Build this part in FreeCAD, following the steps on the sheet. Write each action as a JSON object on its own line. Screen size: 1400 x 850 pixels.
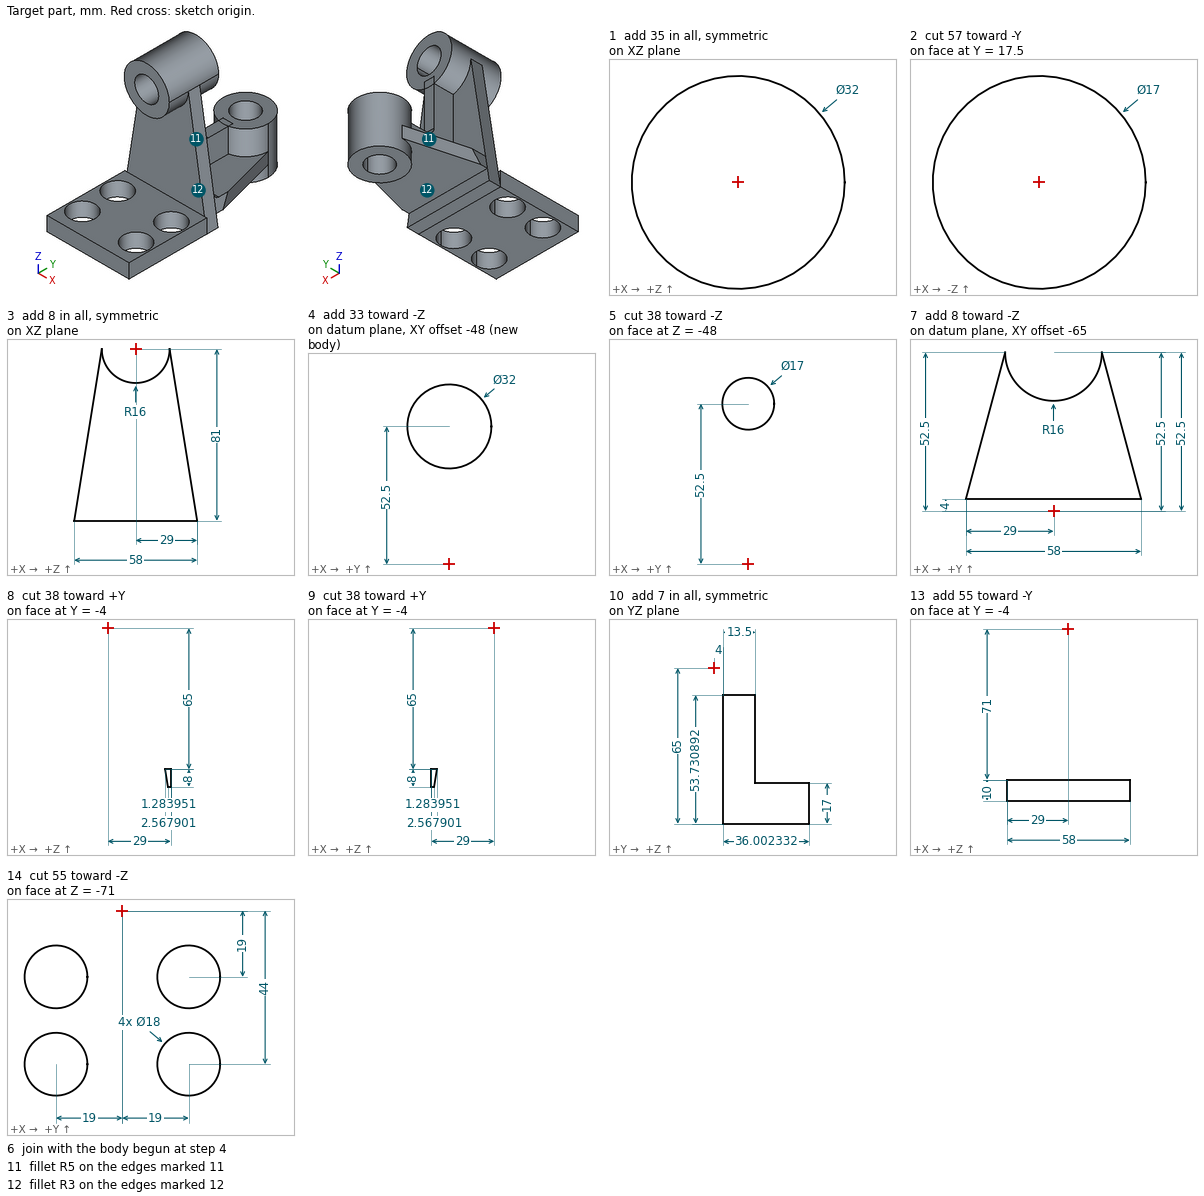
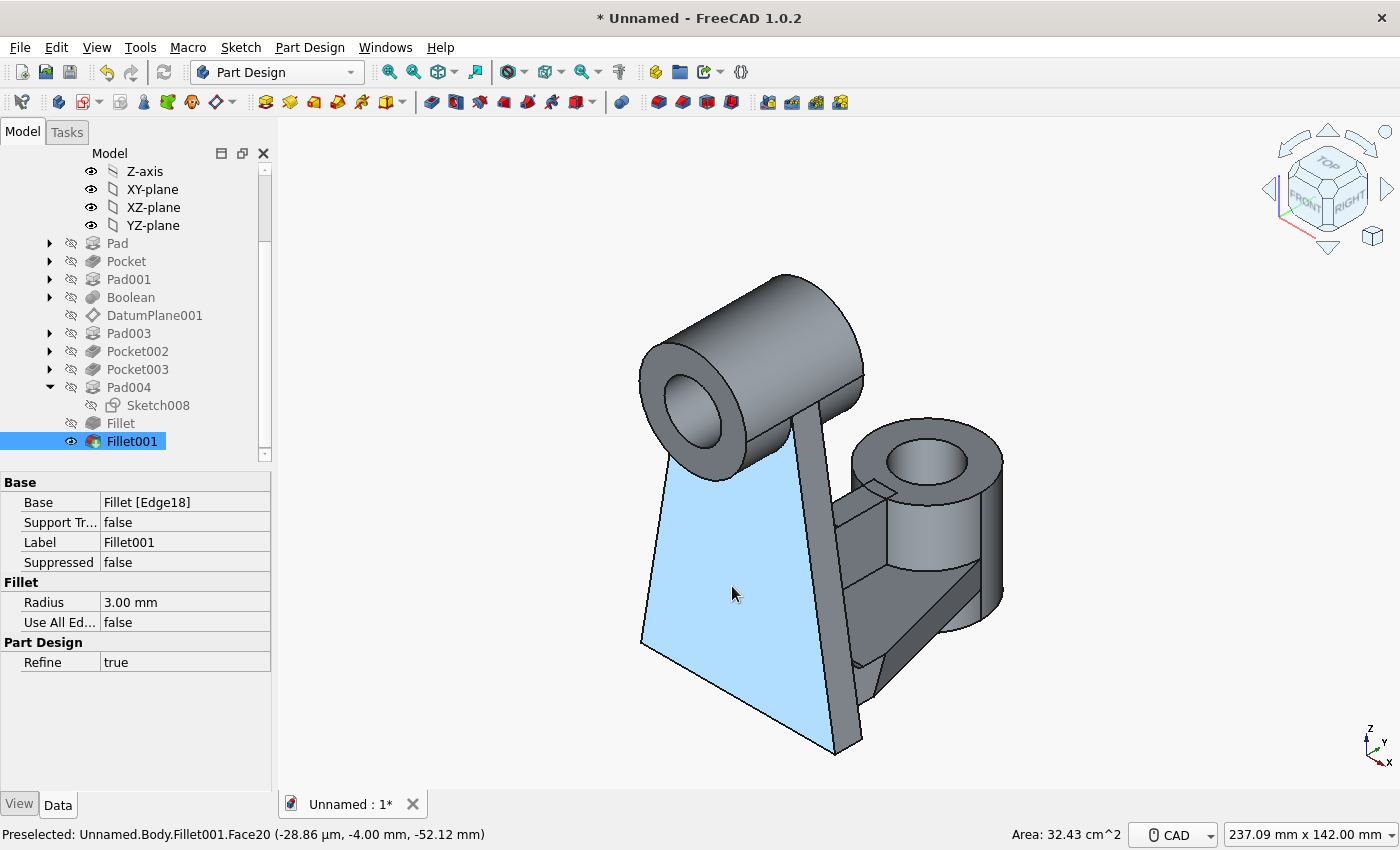
{"action": "left_click", "coordinate": [84, 102]}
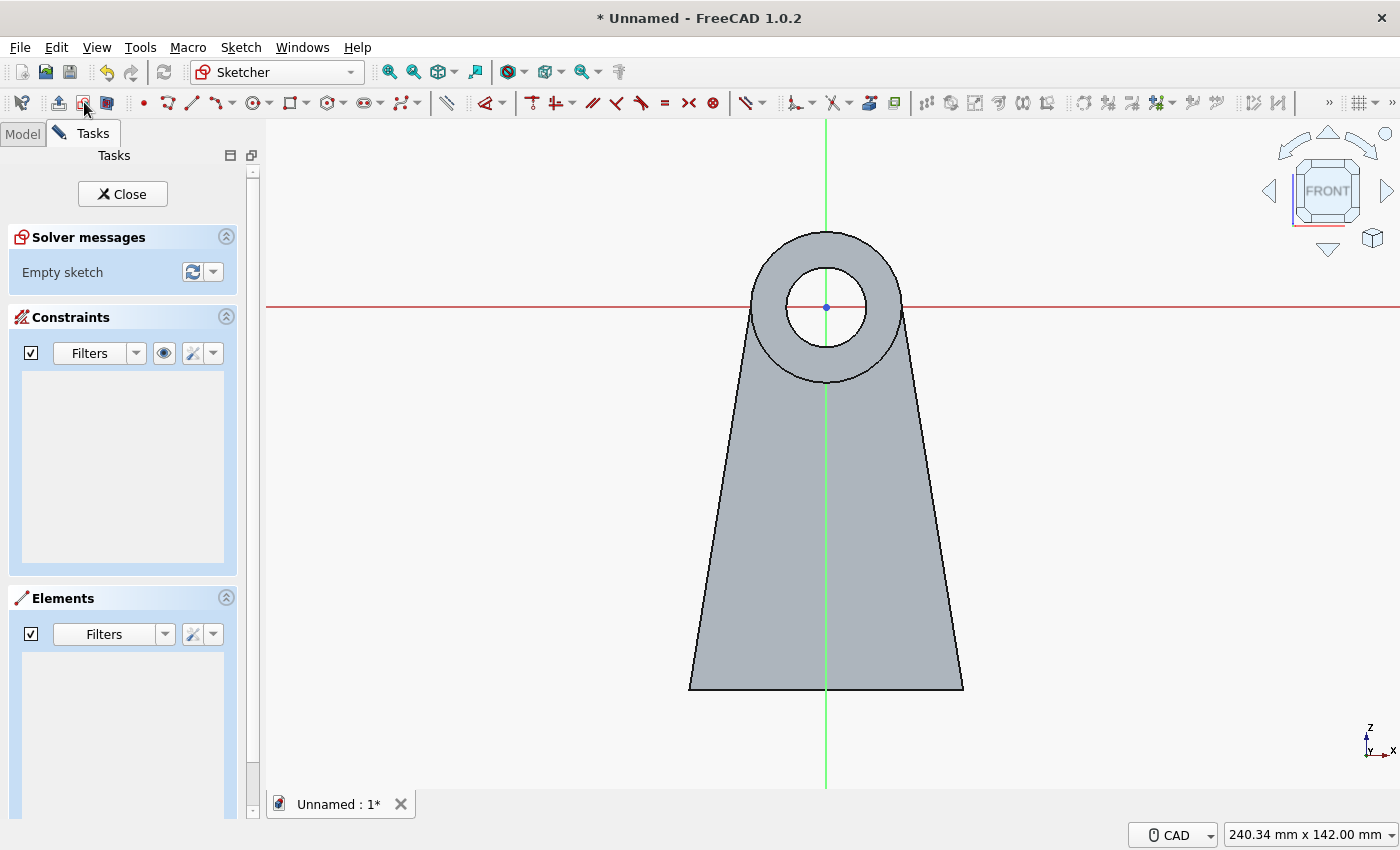
{"action": "key", "text": "g r"}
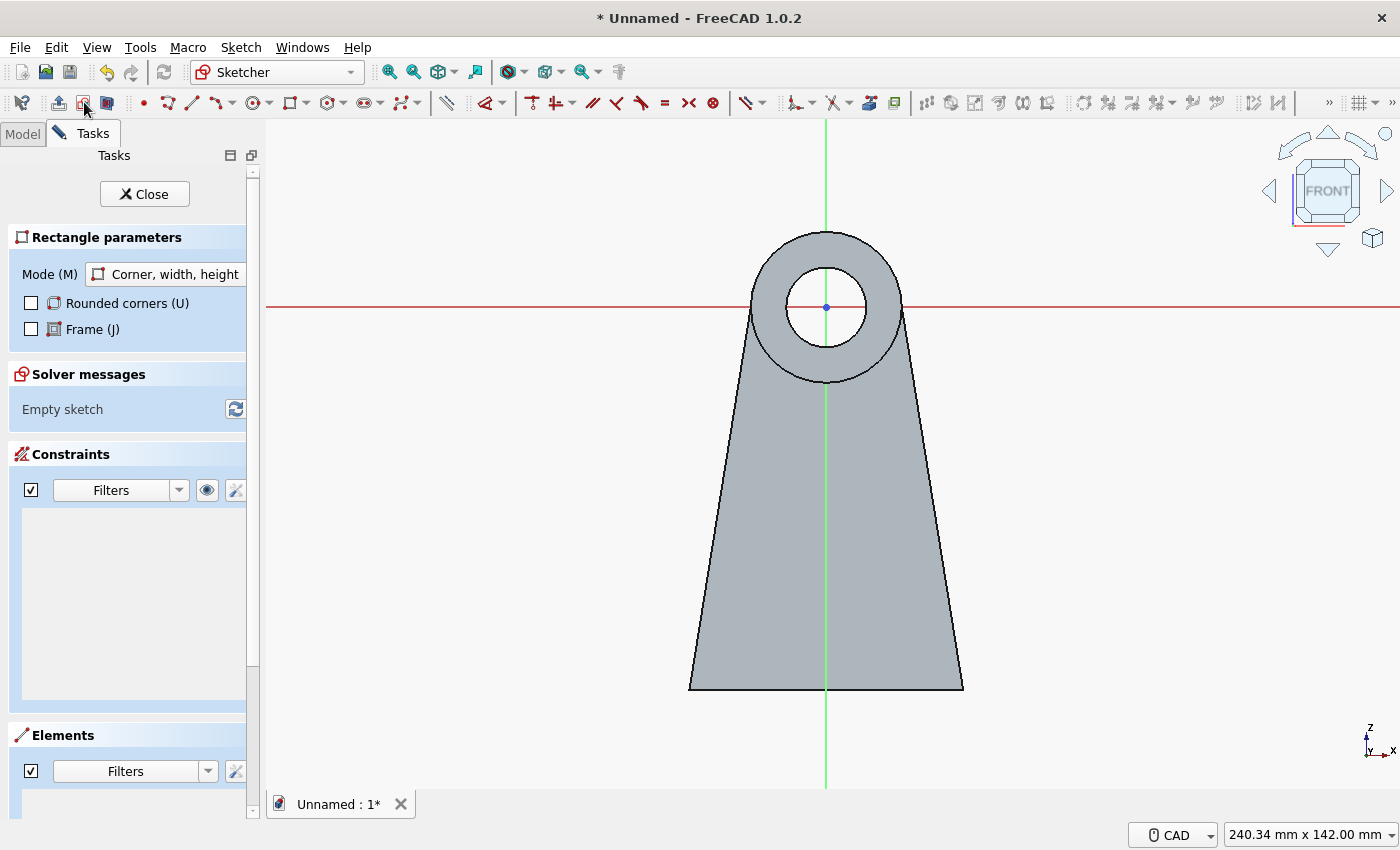
{"action": "left_click", "coordinate": [689, 642]}
{"action": "left_click", "coordinate": [963, 690]}
{"action": "key", "text": "Escape"}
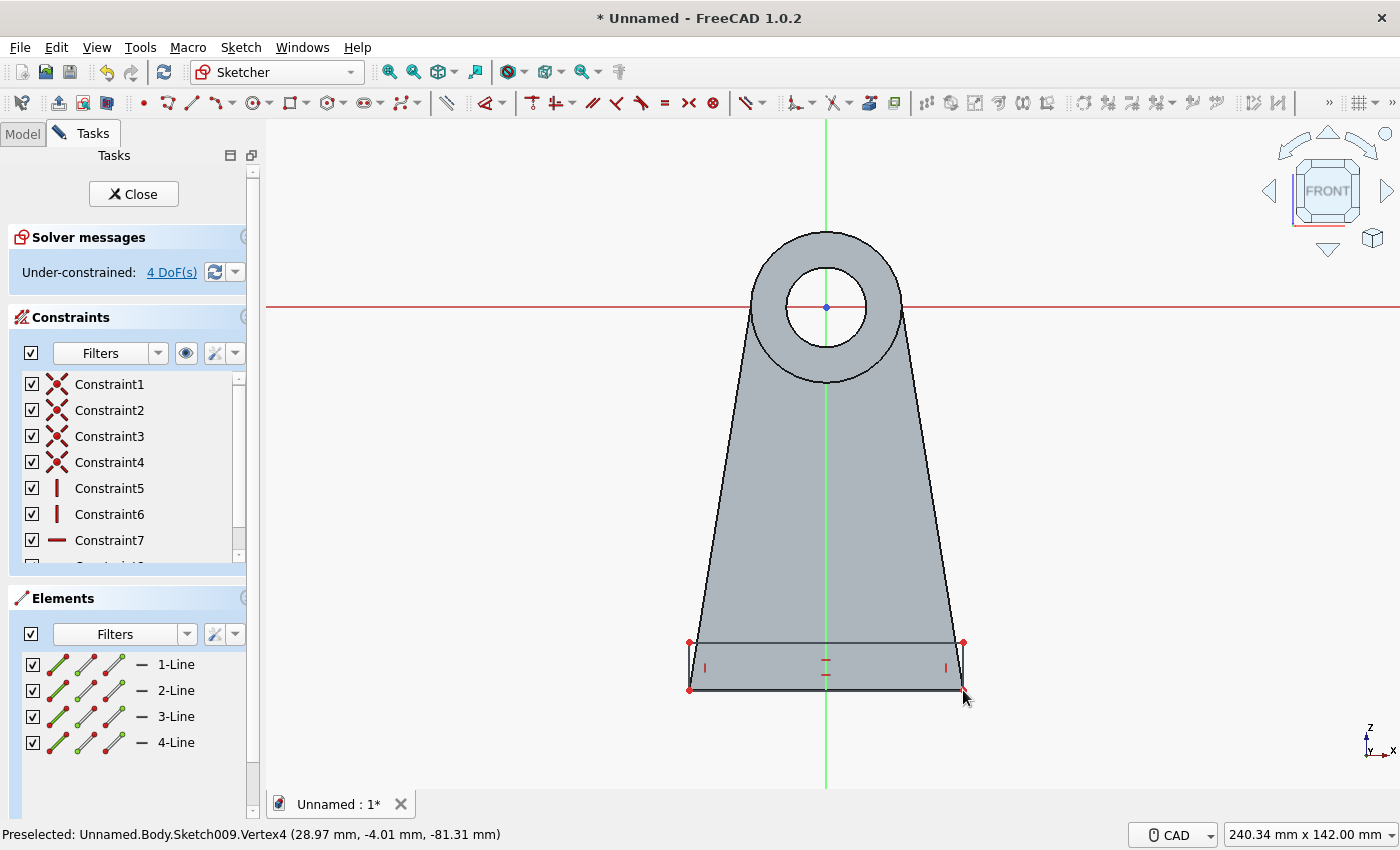
{"action": "left_click", "coordinate": [486, 104]}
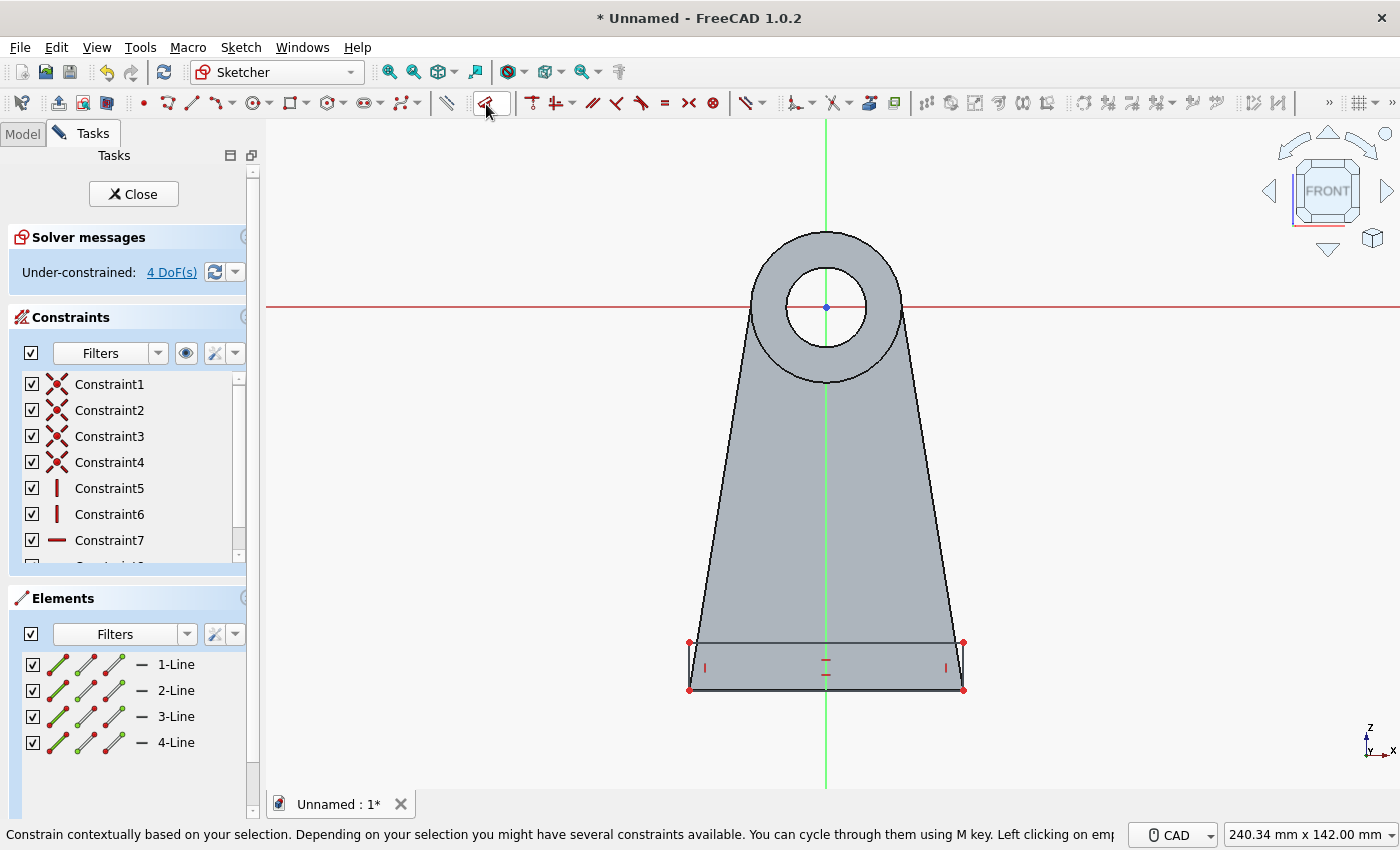
{"action": "left_click", "coordinate": [689, 657]}
{"action": "left_click", "coordinate": [655, 667]}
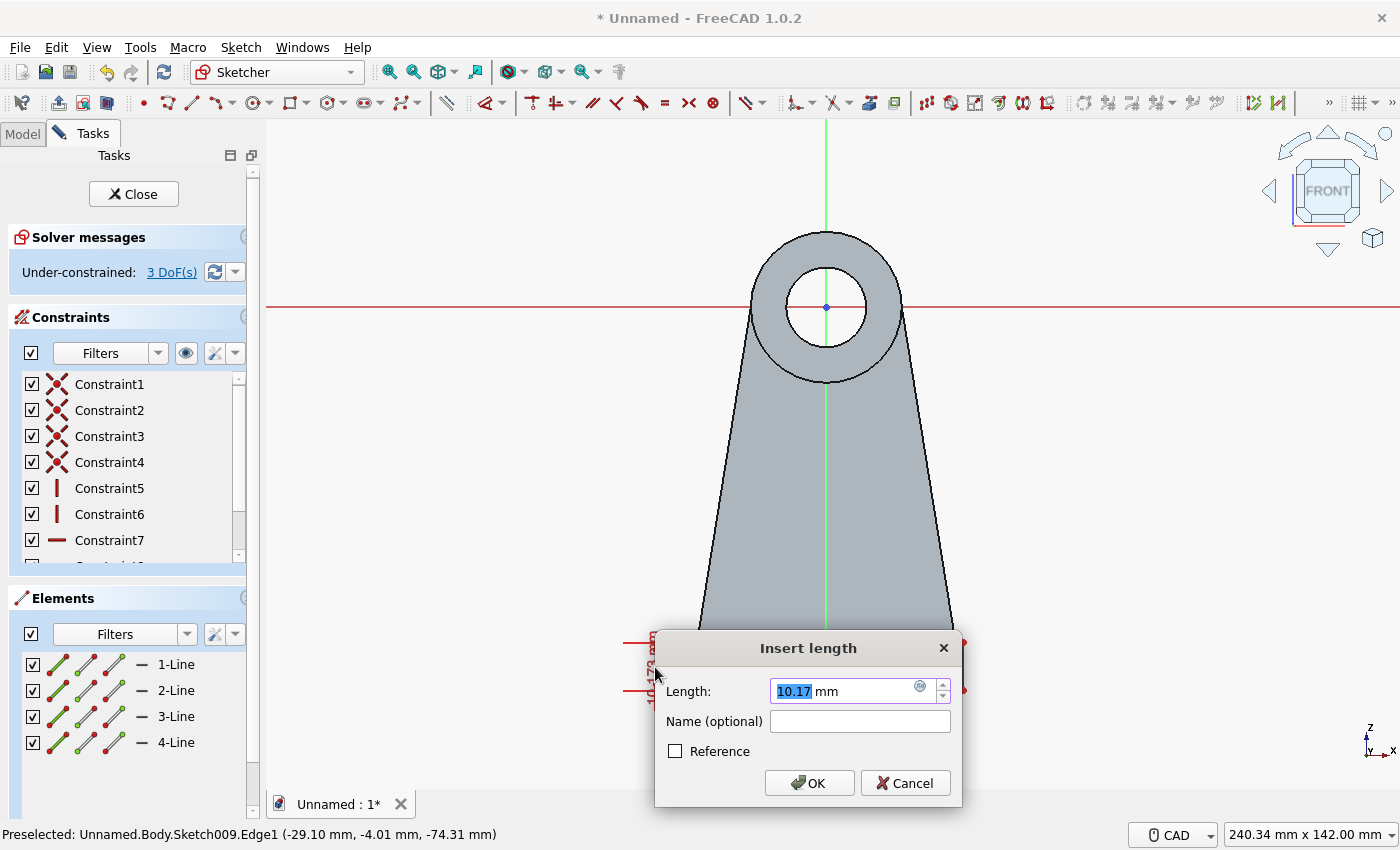
{"action": "type", "text": "10"}
{"action": "key", "text": "Return"}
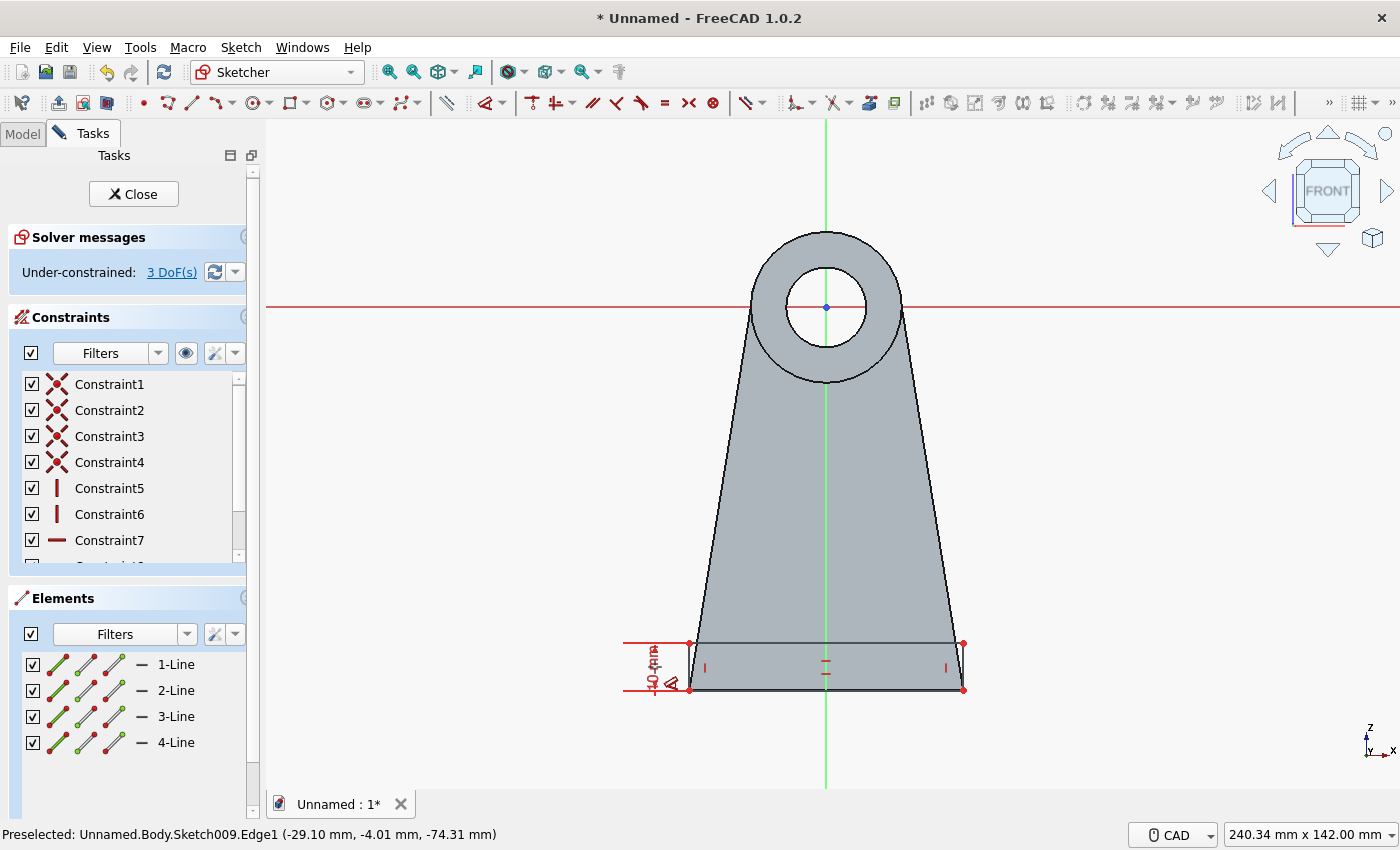
{"action": "left_click", "coordinate": [771, 691]}
{"action": "left_click", "coordinate": [763, 725]}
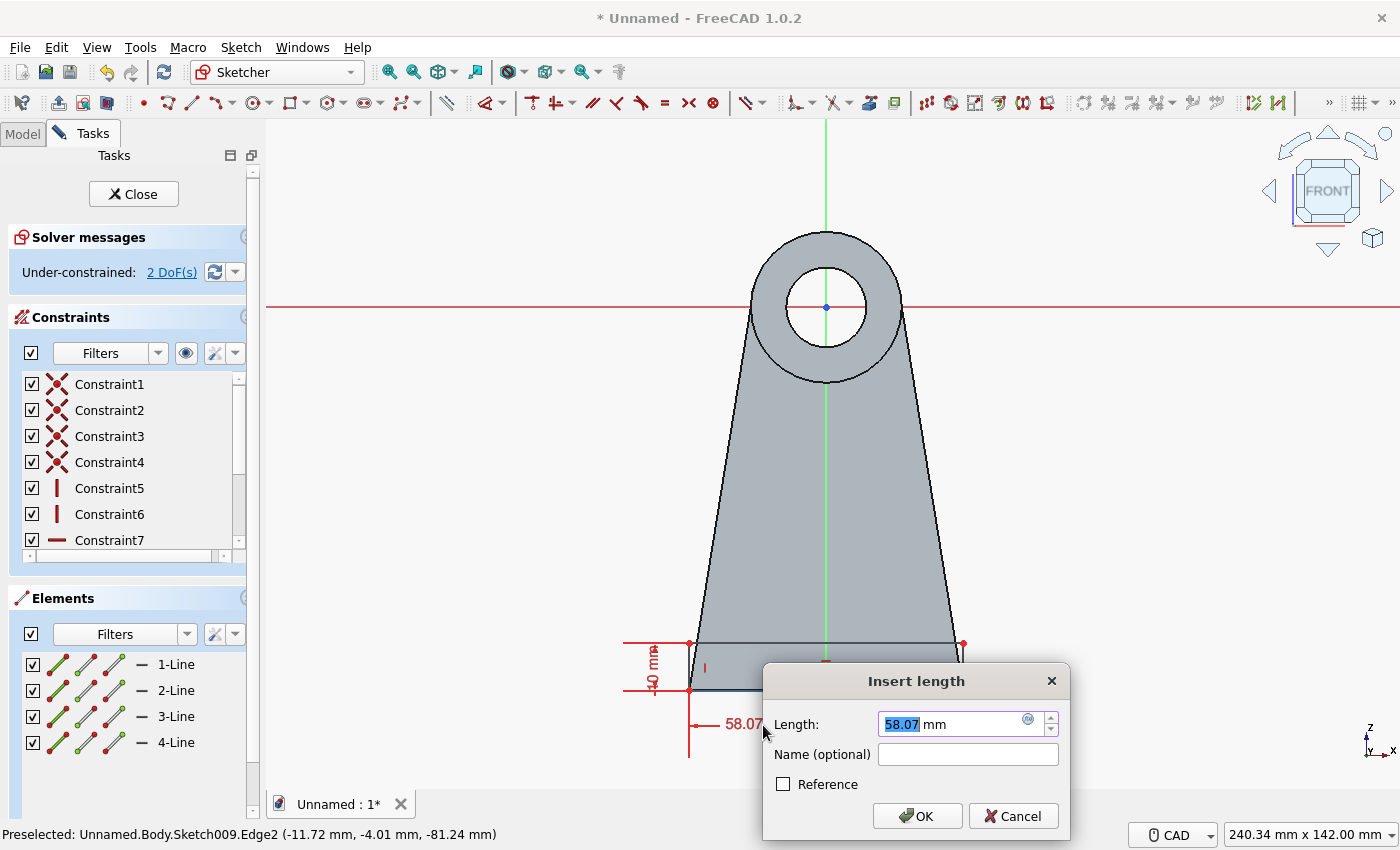
{"action": "type", "text": "58"}
{"action": "key", "text": "Return"}